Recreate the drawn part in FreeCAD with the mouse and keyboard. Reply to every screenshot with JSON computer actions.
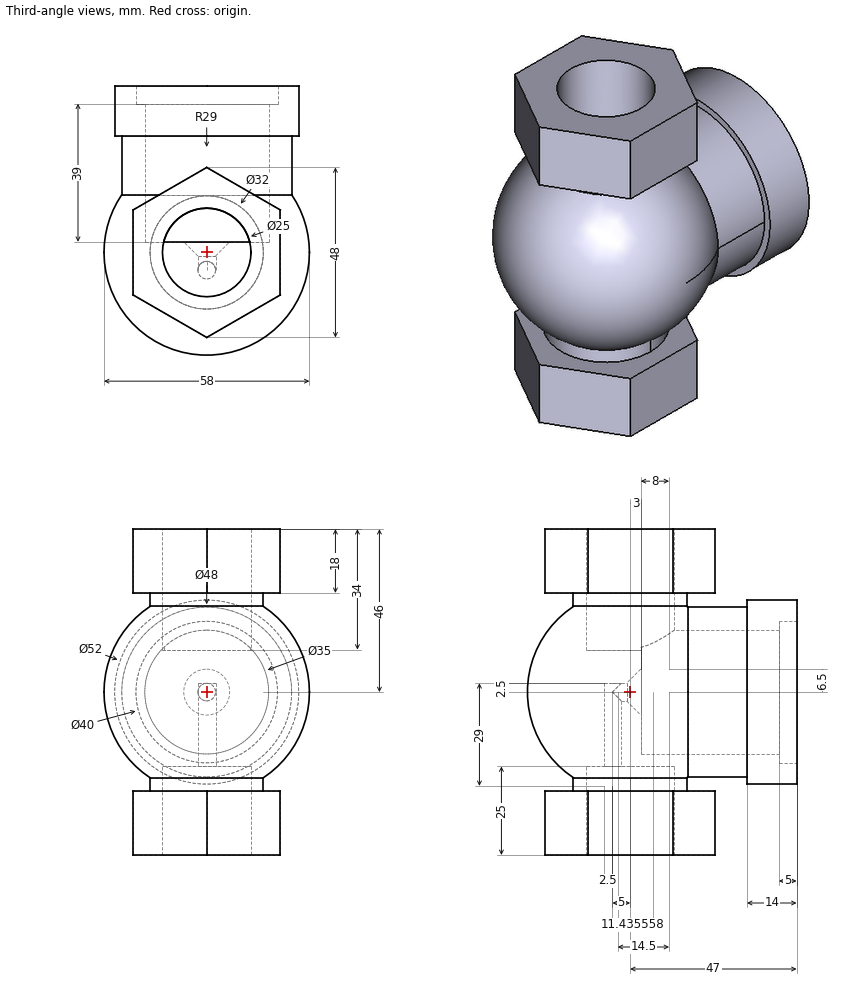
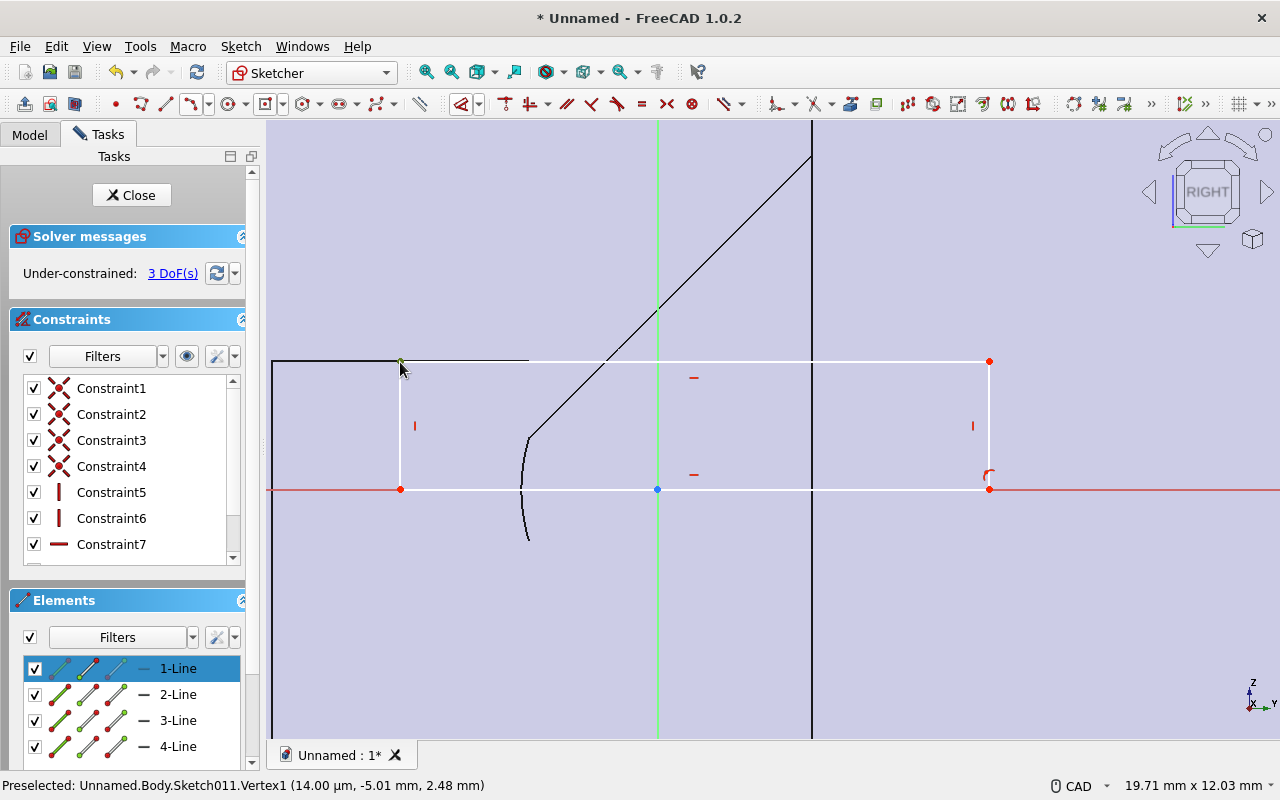
{"action": "key", "text": "l"}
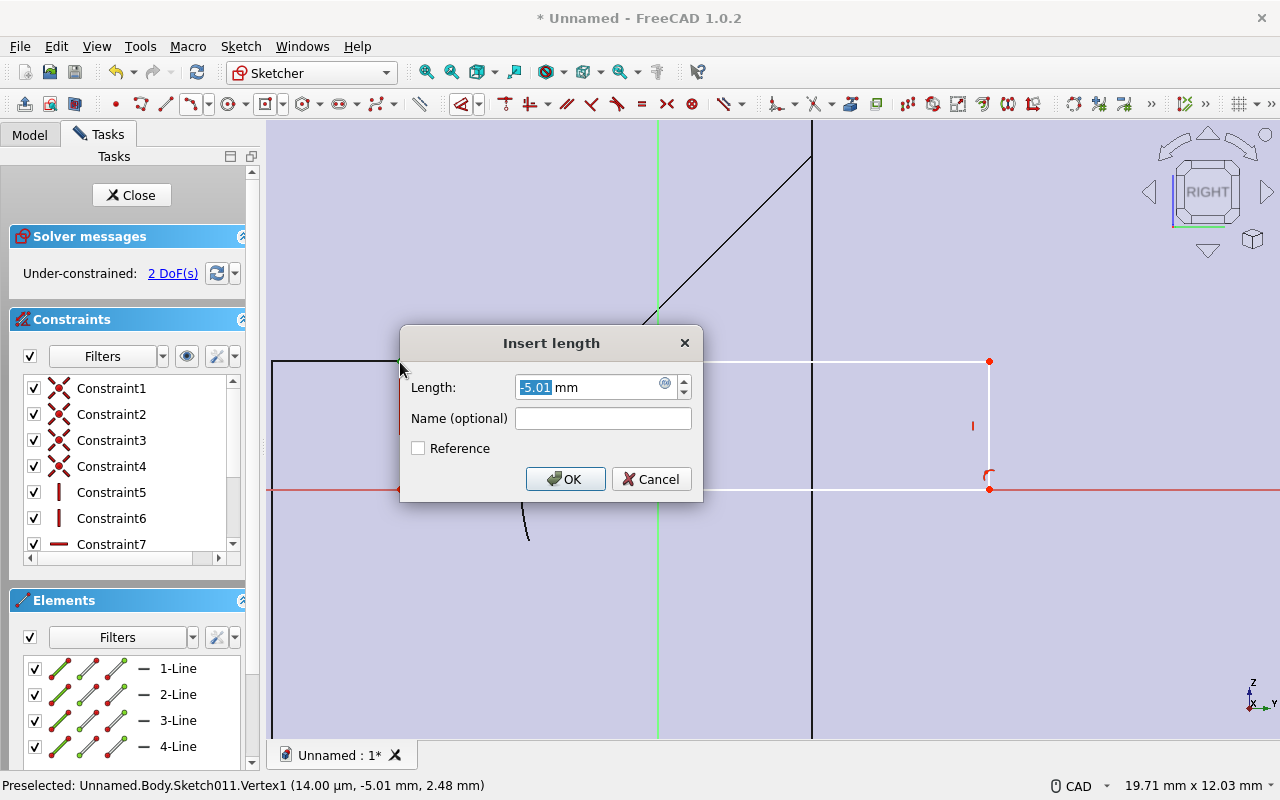
{"action": "type", "text": "-5"}
{"action": "key", "text": "Return"}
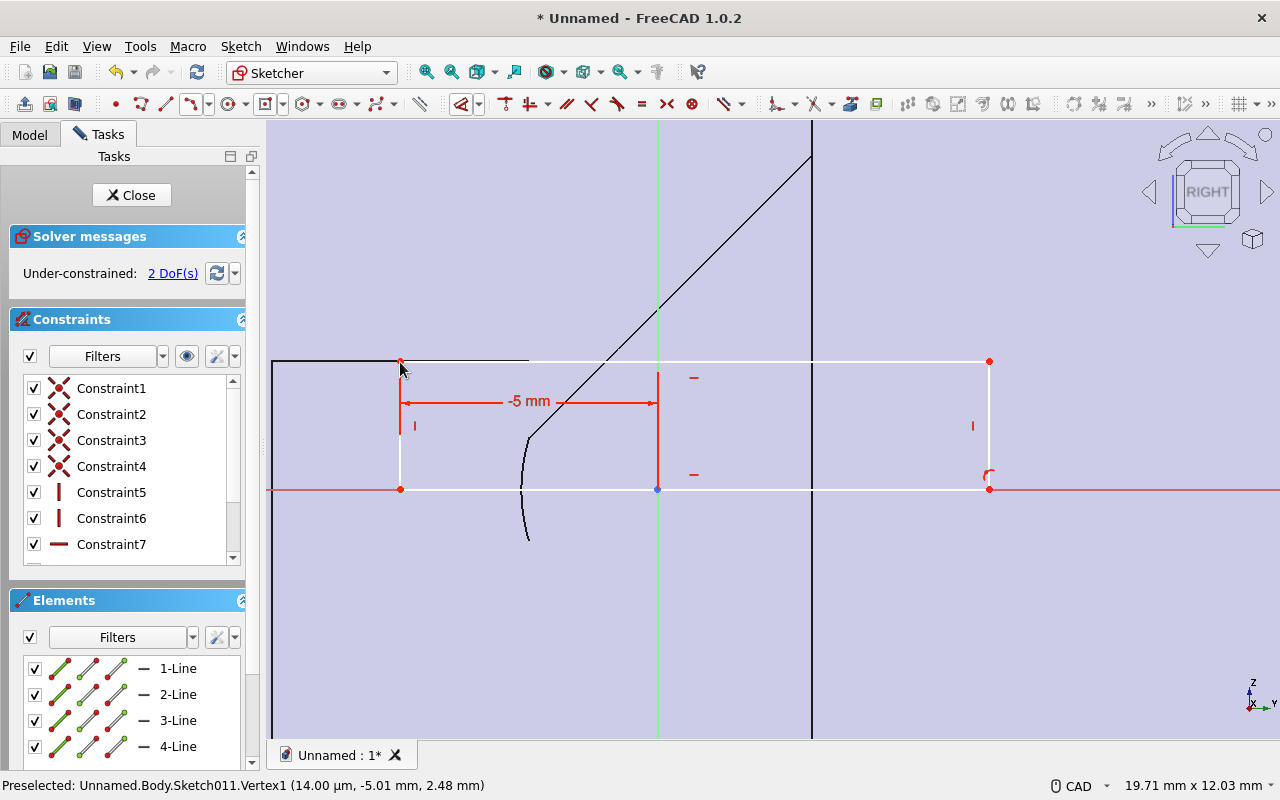
{"action": "left_click", "coordinate": [400, 400]}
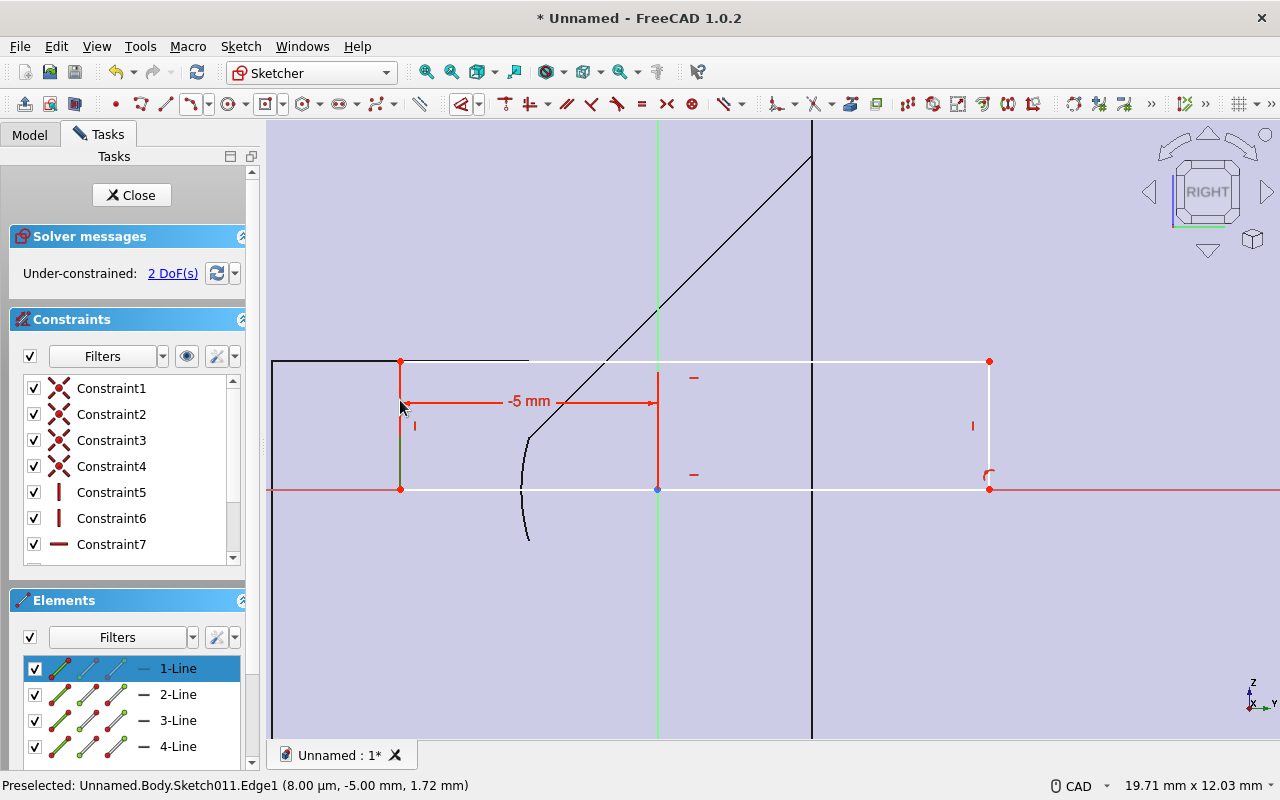
{"action": "left_click", "coordinate": [478, 104]}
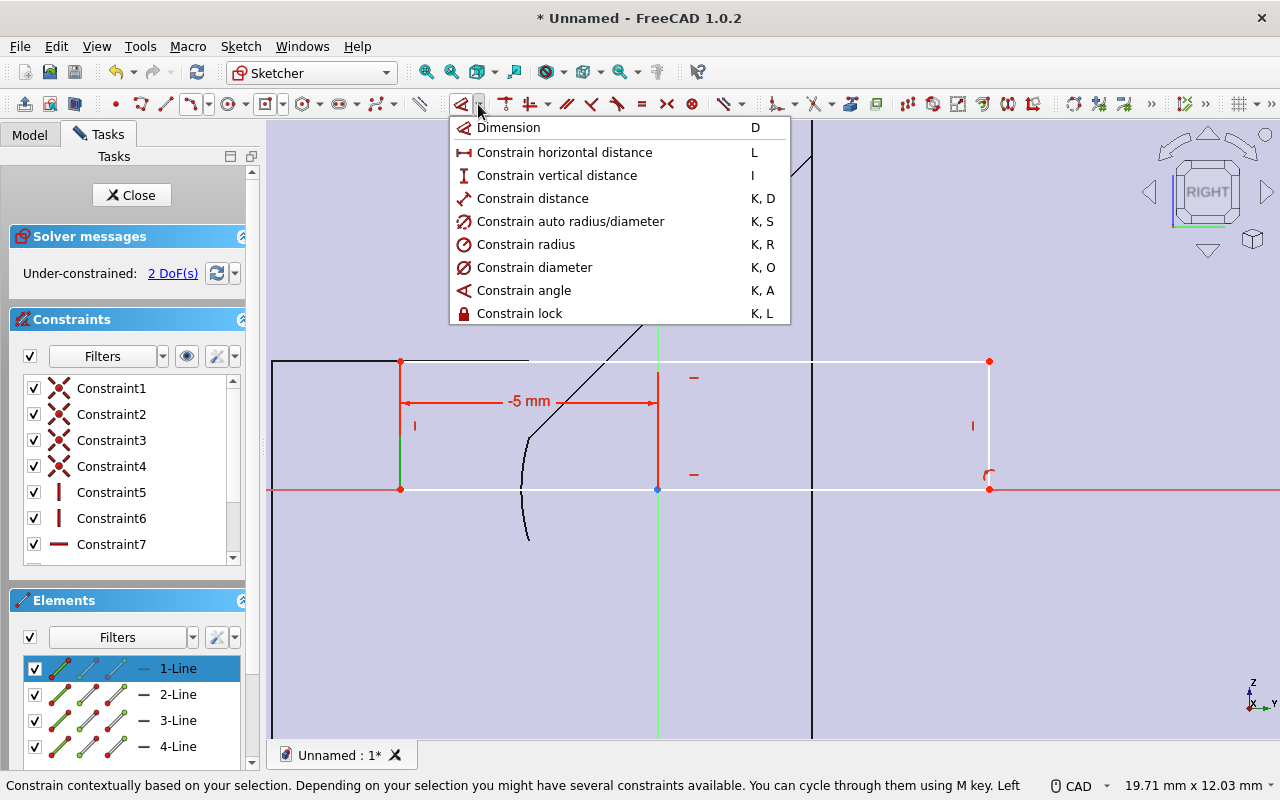
{"action": "left_click", "coordinate": [620, 176]}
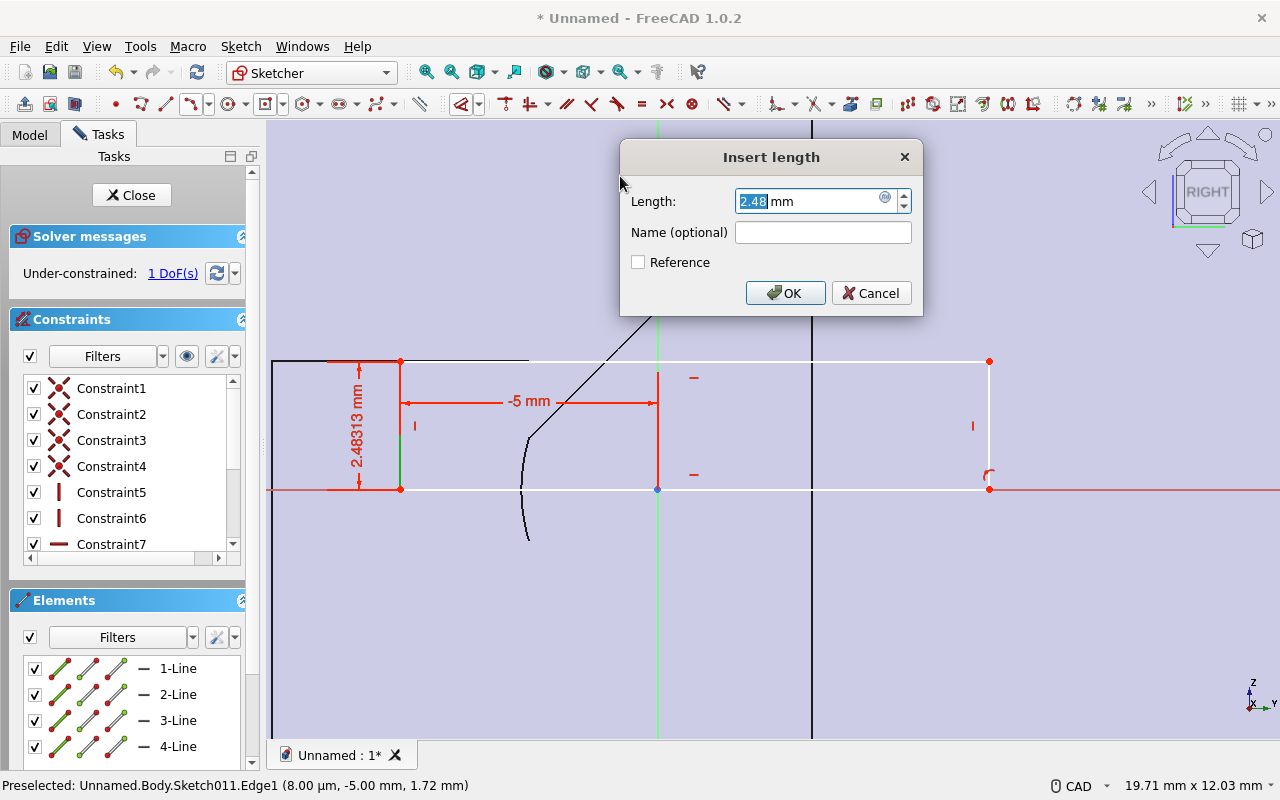
{"action": "type", "text": "2.5"}
{"action": "key", "text": "Return"}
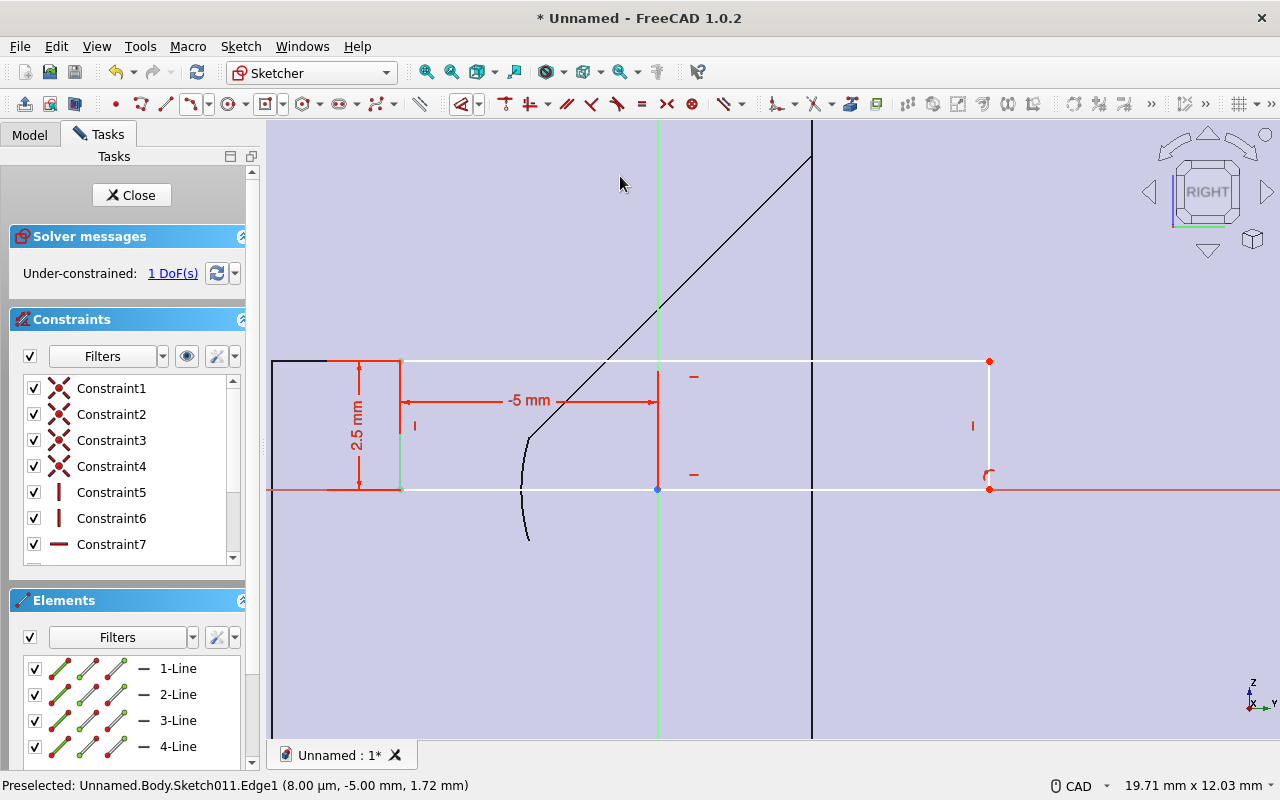
{"action": "left_click", "coordinate": [577, 490]}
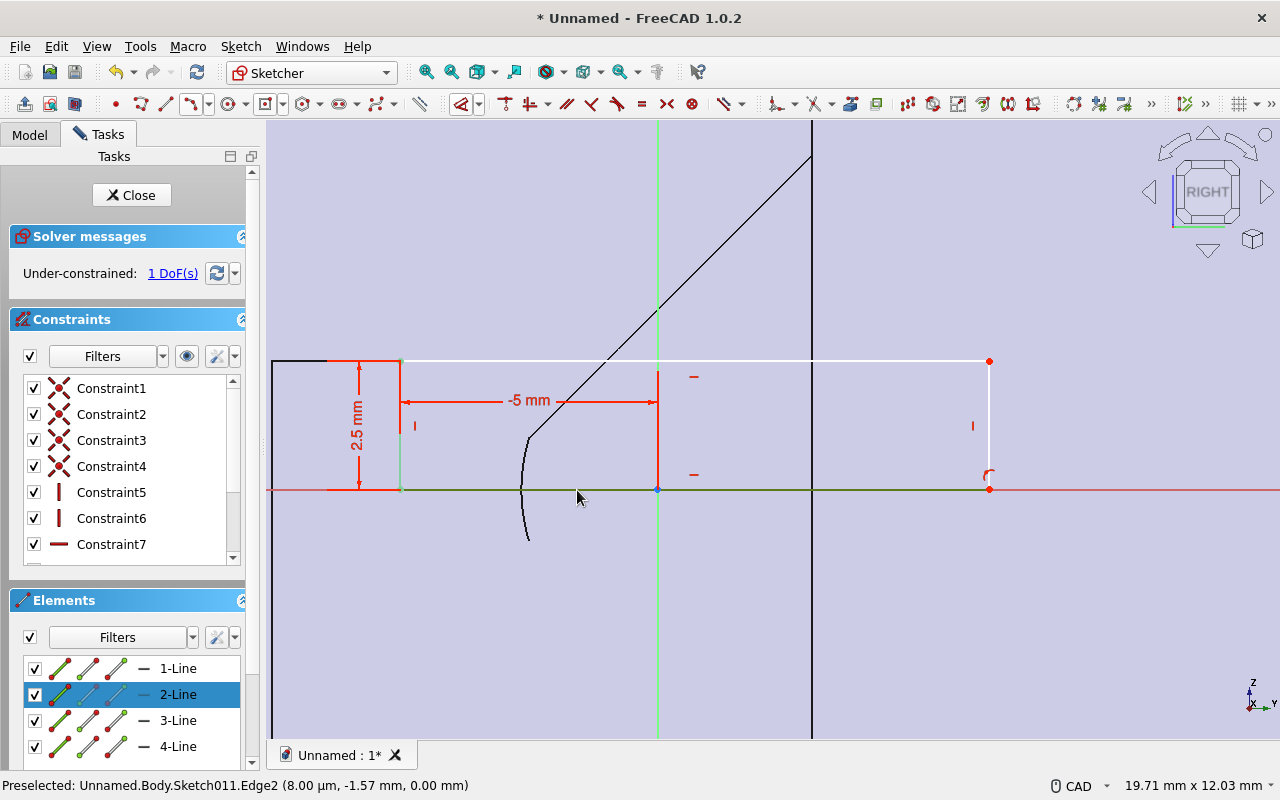
{"action": "left_click", "coordinate": [478, 104]}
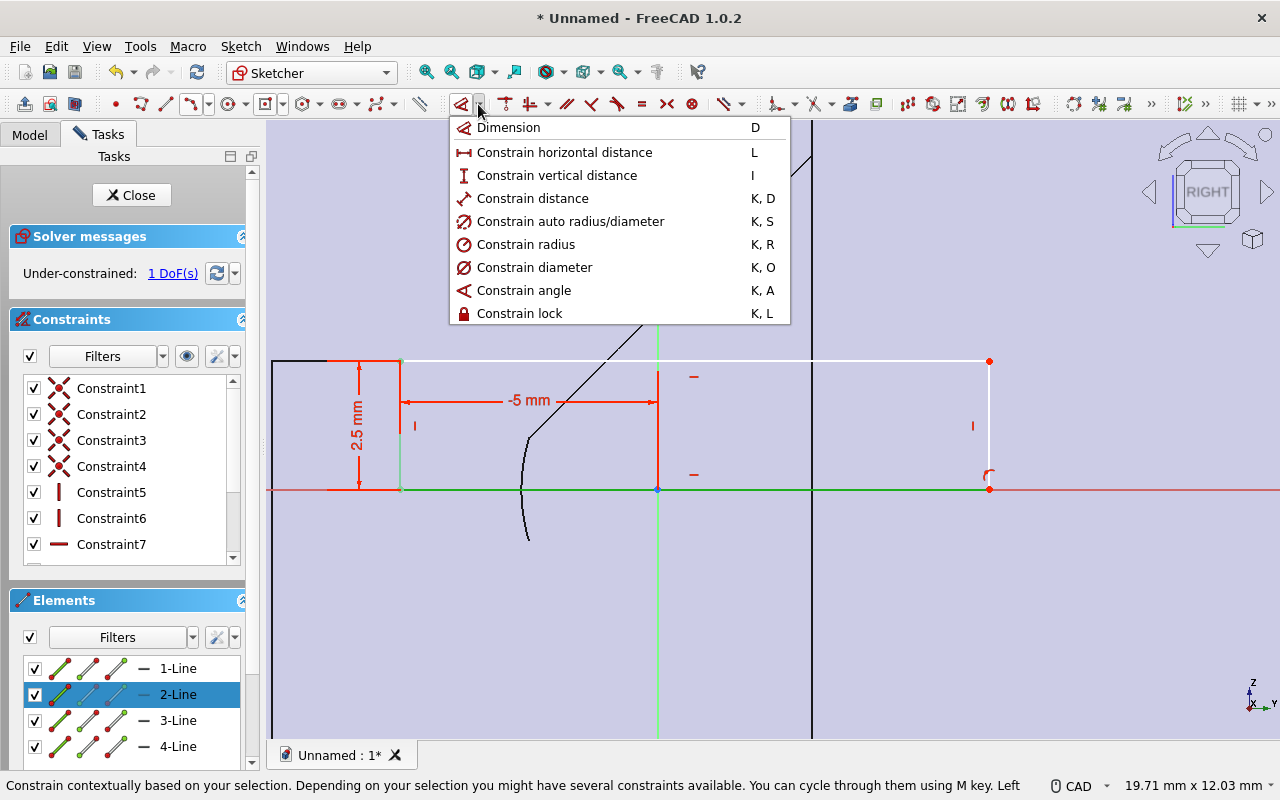
{"action": "left_click", "coordinate": [620, 152]}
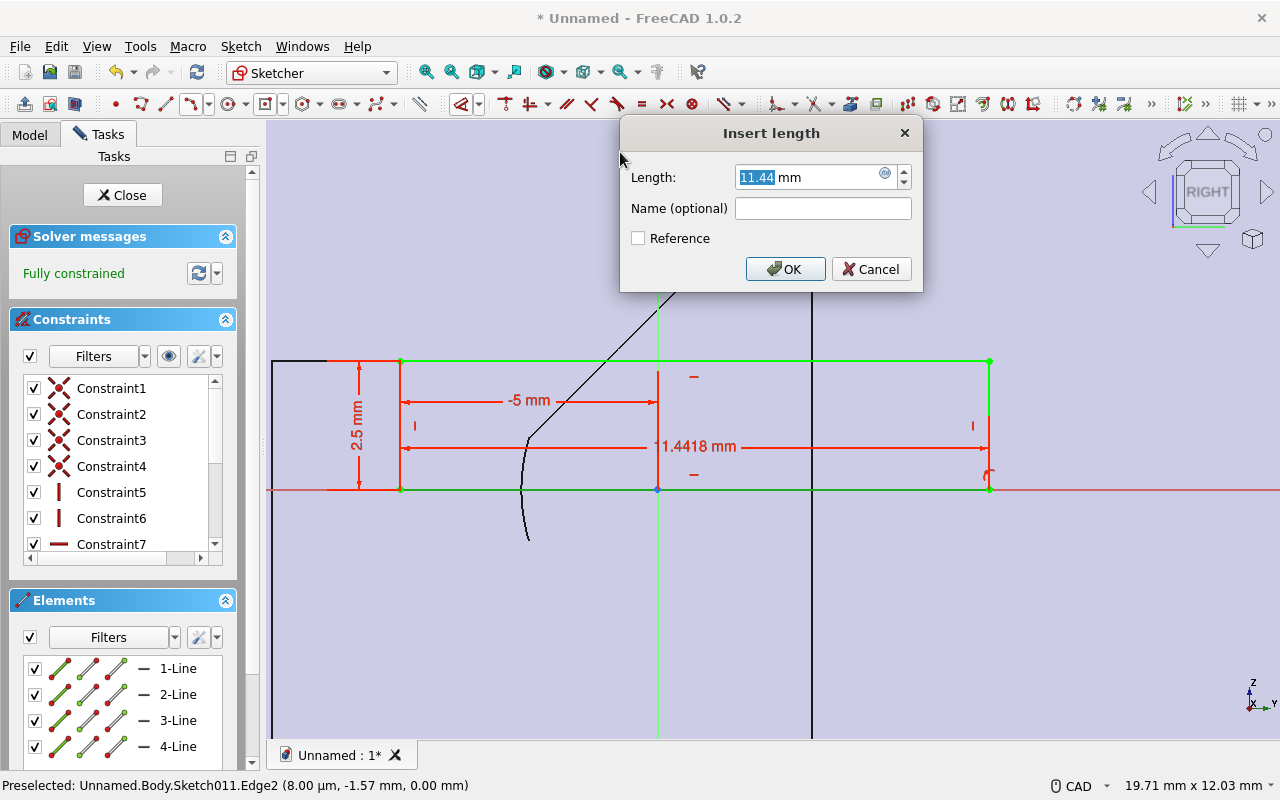
{"action": "type", "text": "11.435558"}
{"action": "key", "text": "Return"}